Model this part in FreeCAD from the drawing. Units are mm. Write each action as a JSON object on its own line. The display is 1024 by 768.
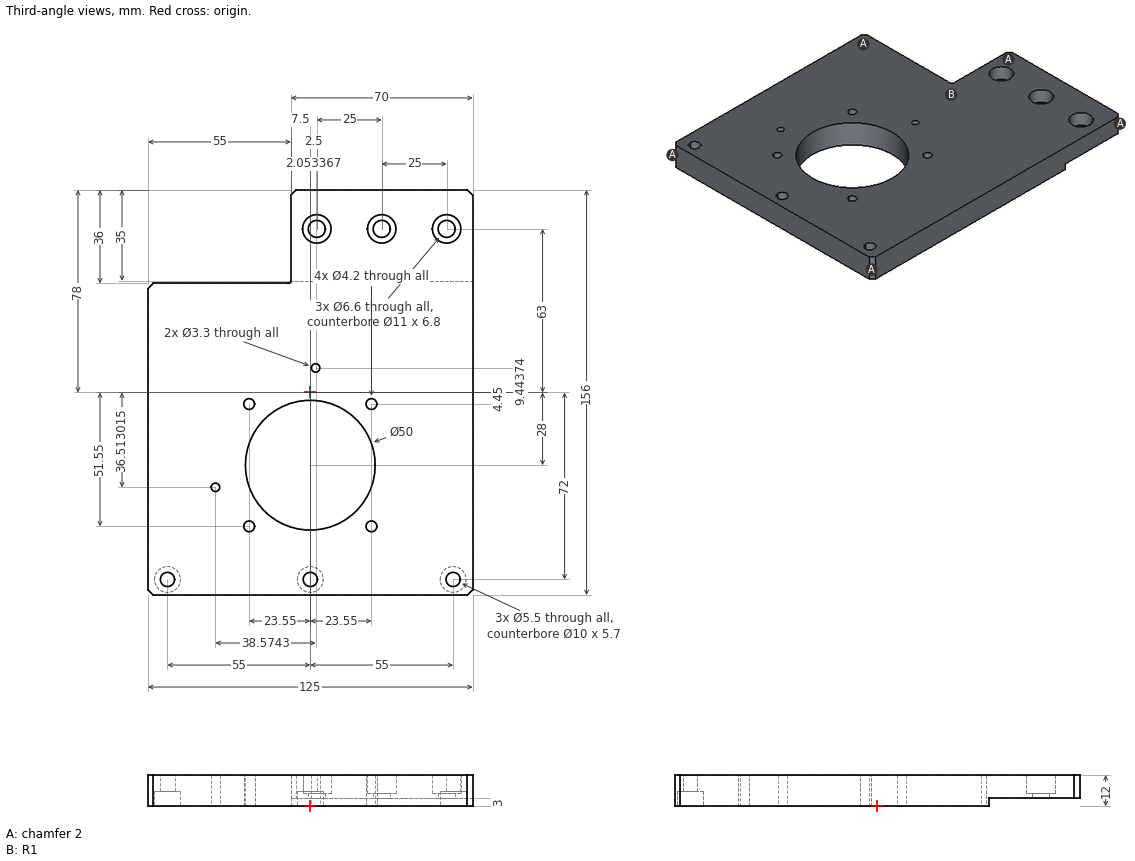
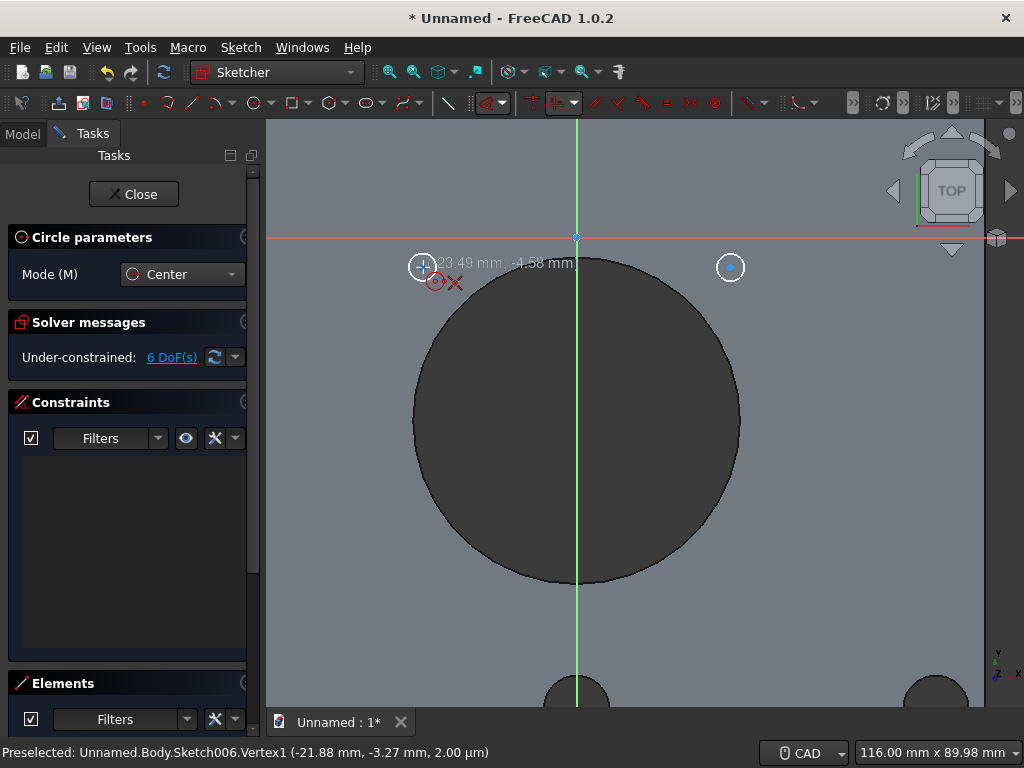
{"action": "scroll", "coordinate": [423, 575], "scroll_direction": "up", "scroll_amount": 3}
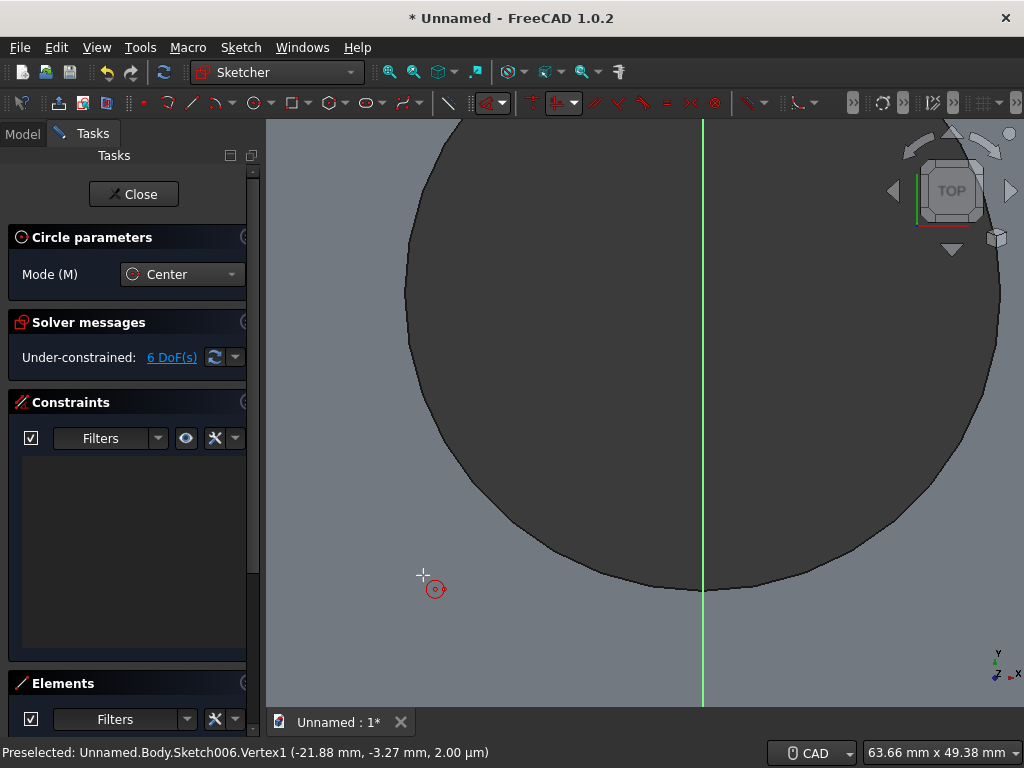
{"action": "left_click", "coordinate": [422, 574]}
{"action": "left_click", "coordinate": [440, 556]}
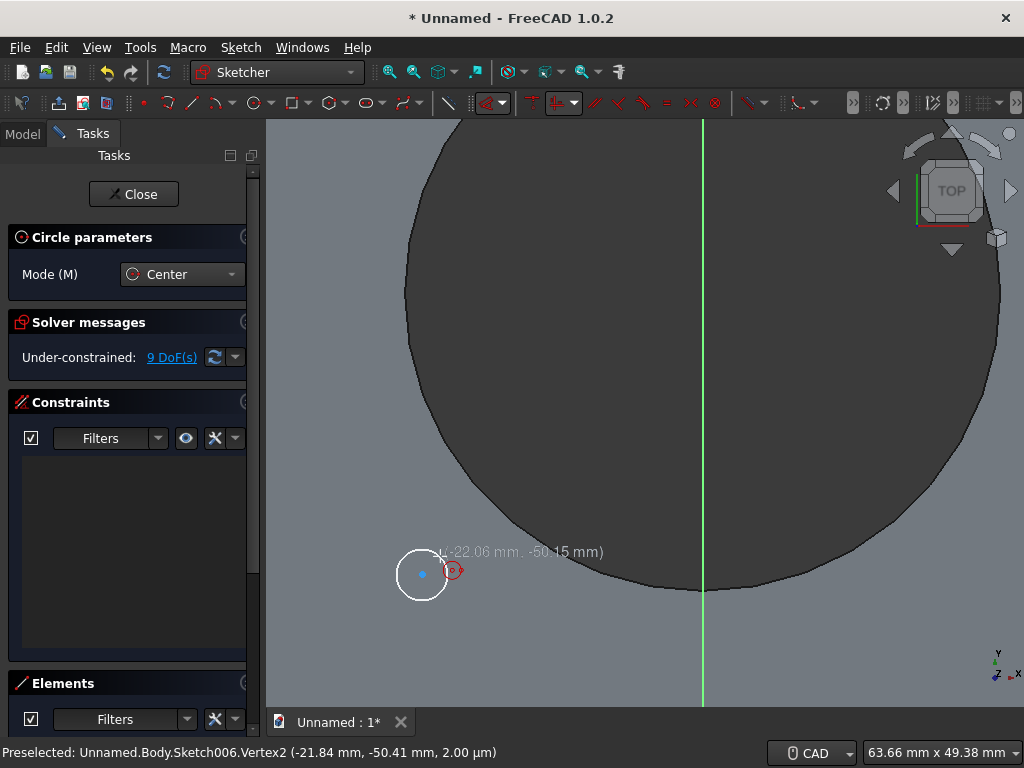
{"action": "scroll", "coordinate": [423, 576], "scroll_direction": "down", "scroll_amount": 3}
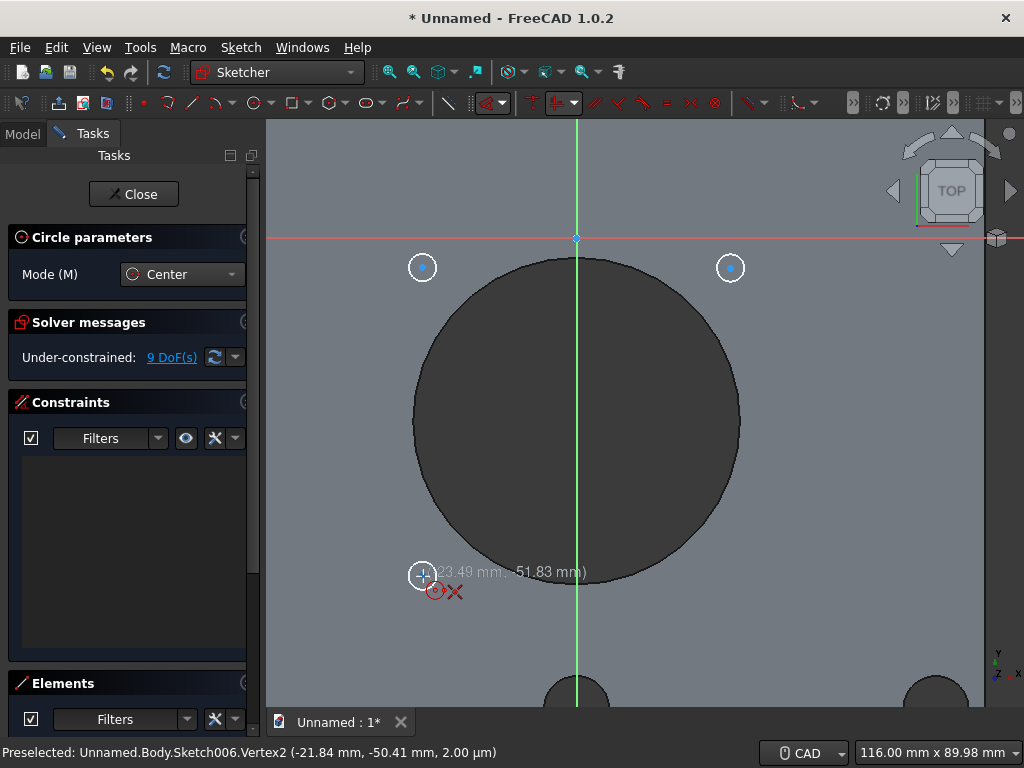
{"action": "scroll", "coordinate": [730, 575], "scroll_direction": "up", "scroll_amount": 3}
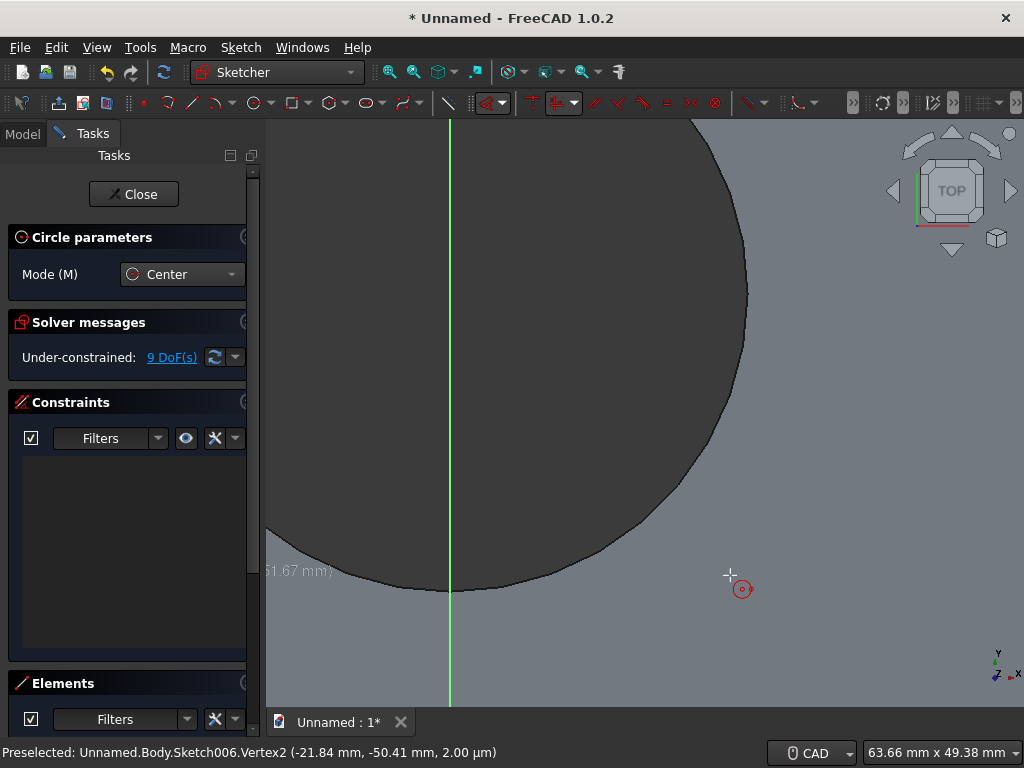
{"action": "left_click", "coordinate": [730, 574]}
{"action": "left_click", "coordinate": [748, 557]}
{"action": "key", "text": "Escape"}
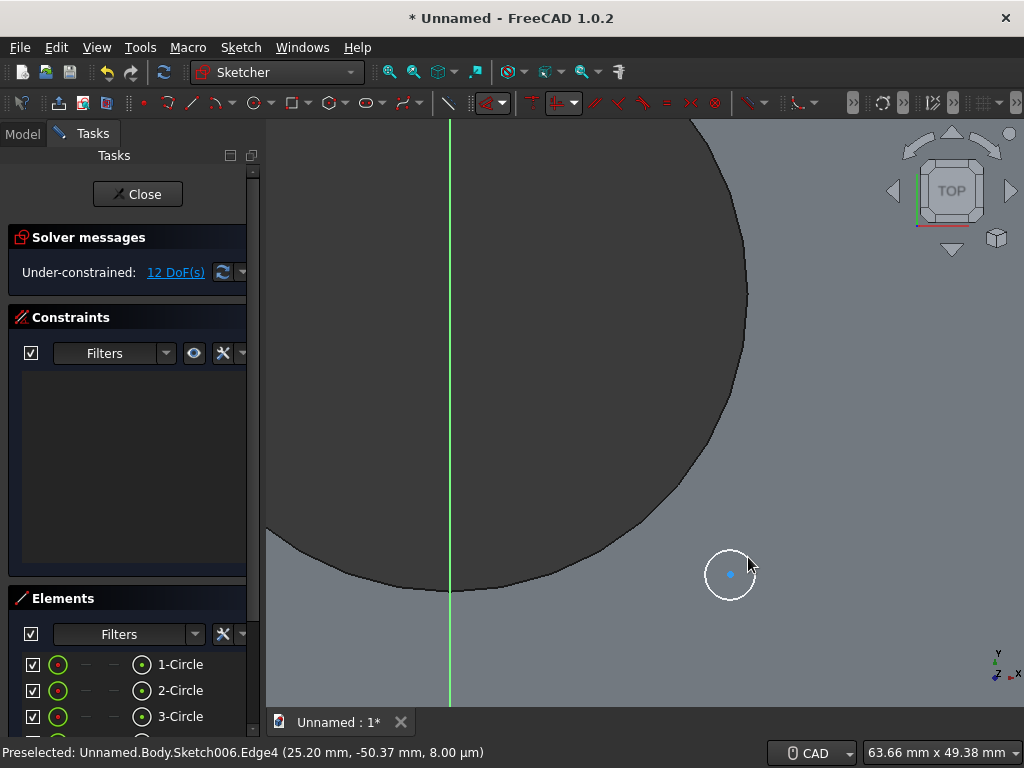
{"action": "scroll", "coordinate": [730, 575], "scroll_direction": "down", "scroll_amount": 3}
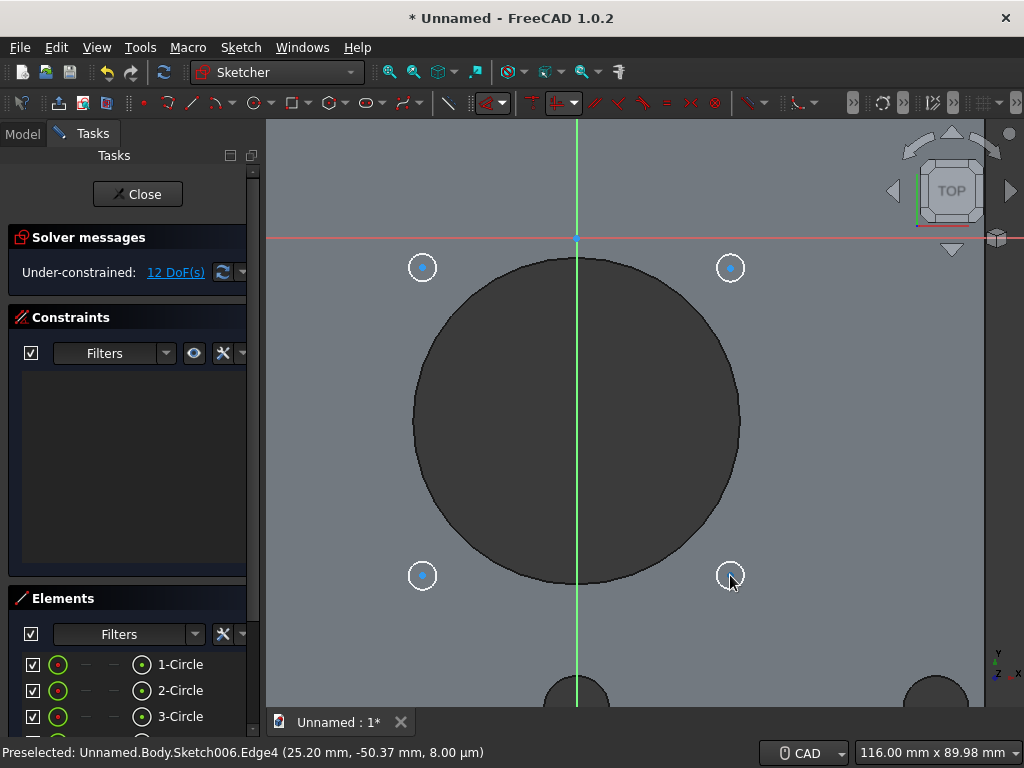
{"action": "left_click", "coordinate": [740, 258]}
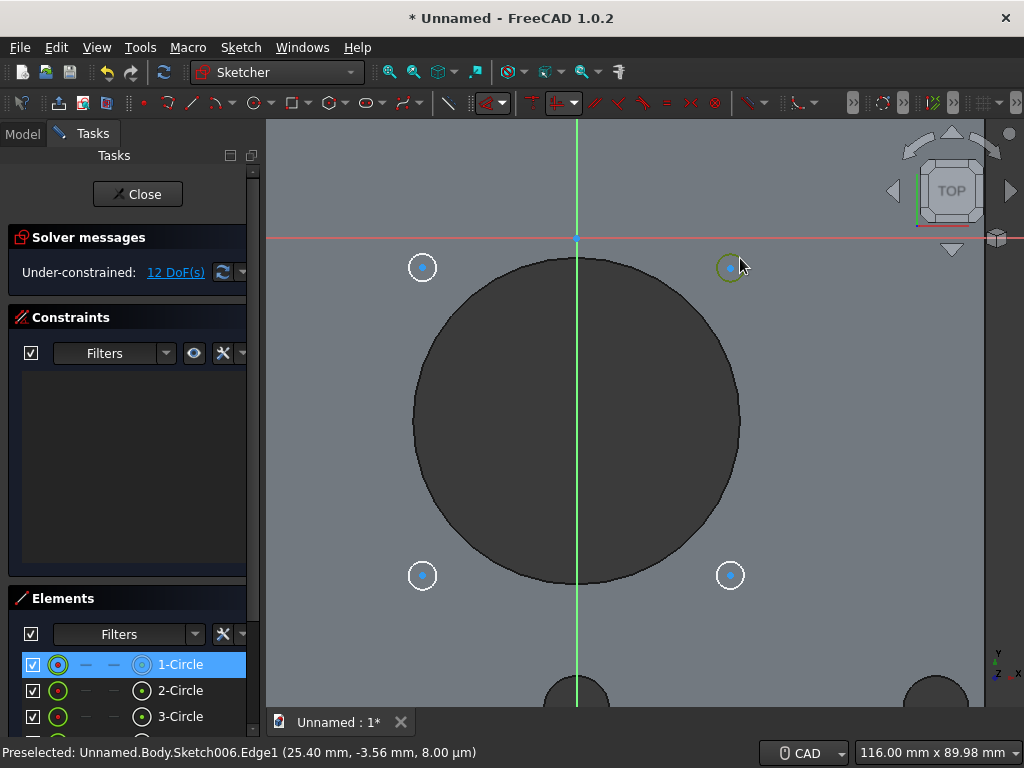
{"action": "left_click", "coordinate": [432, 258]}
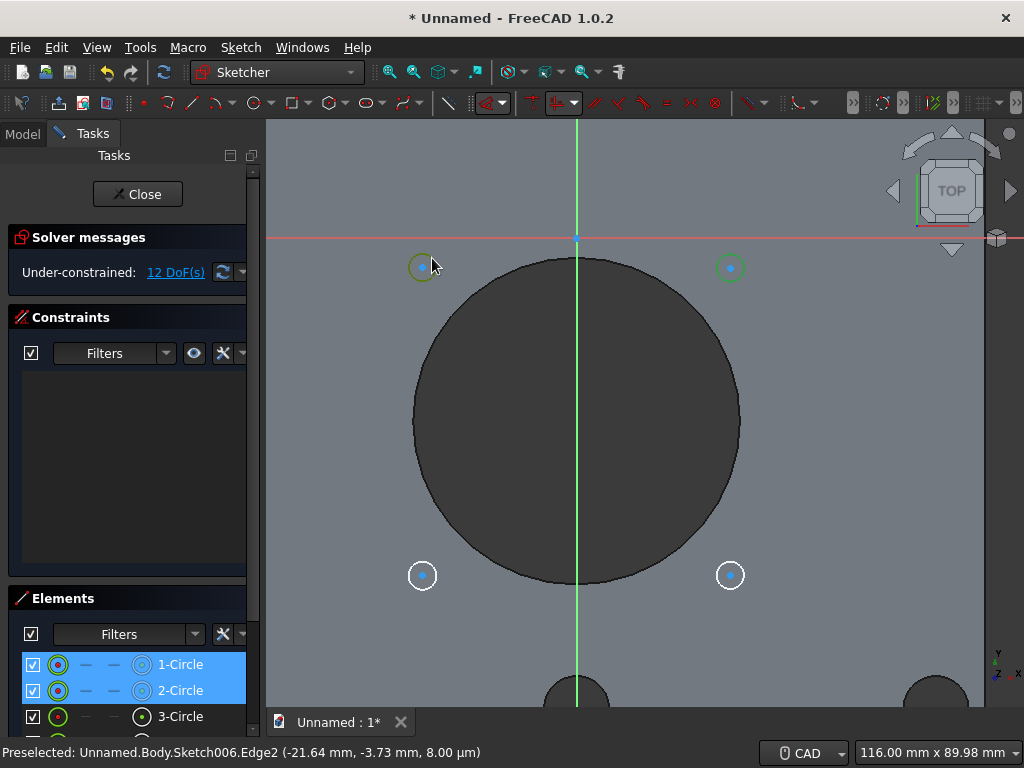
{"action": "left_click", "coordinate": [432, 566]}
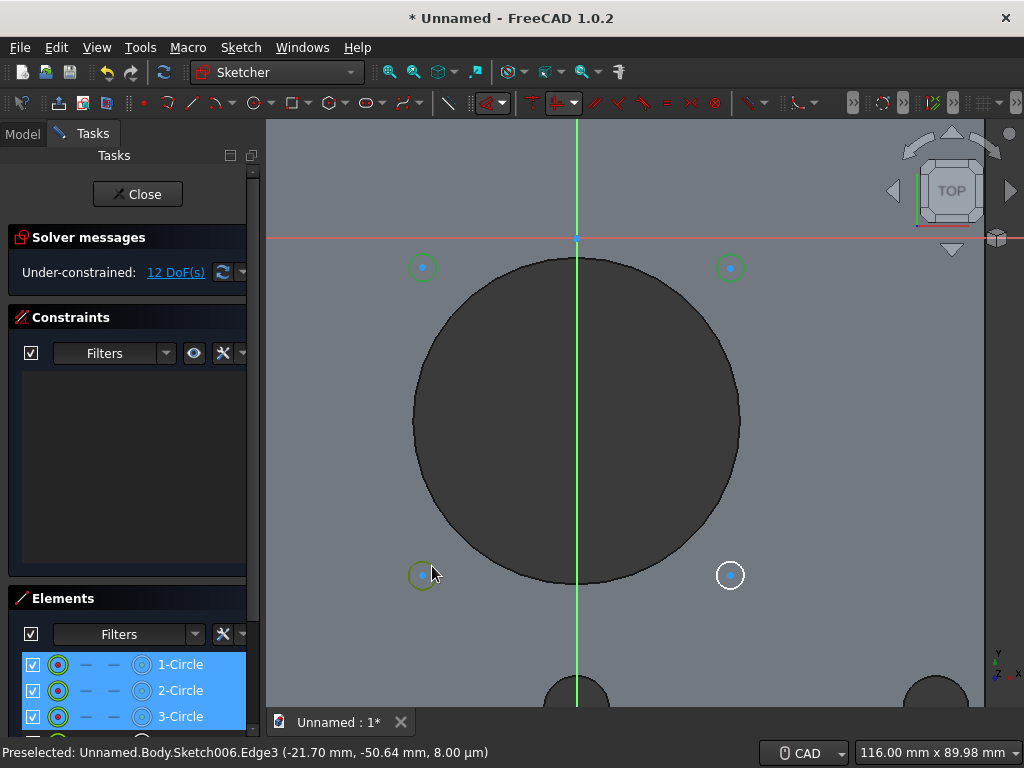
{"action": "left_click", "coordinate": [740, 566]}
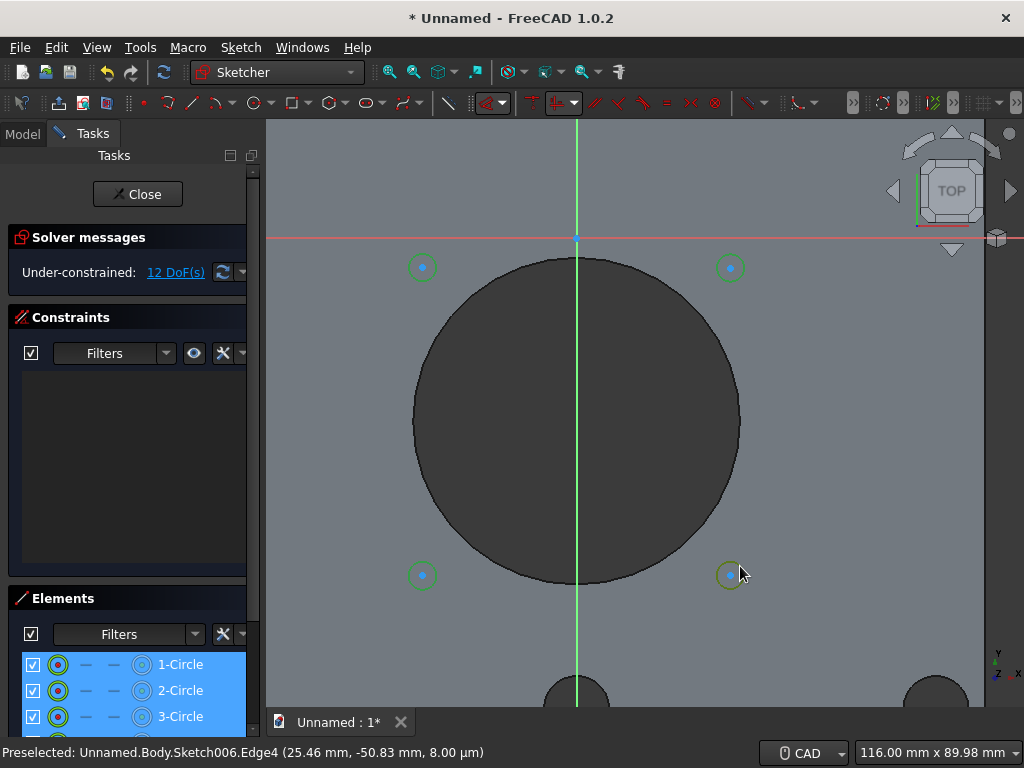
{"action": "left_click", "coordinate": [668, 104]}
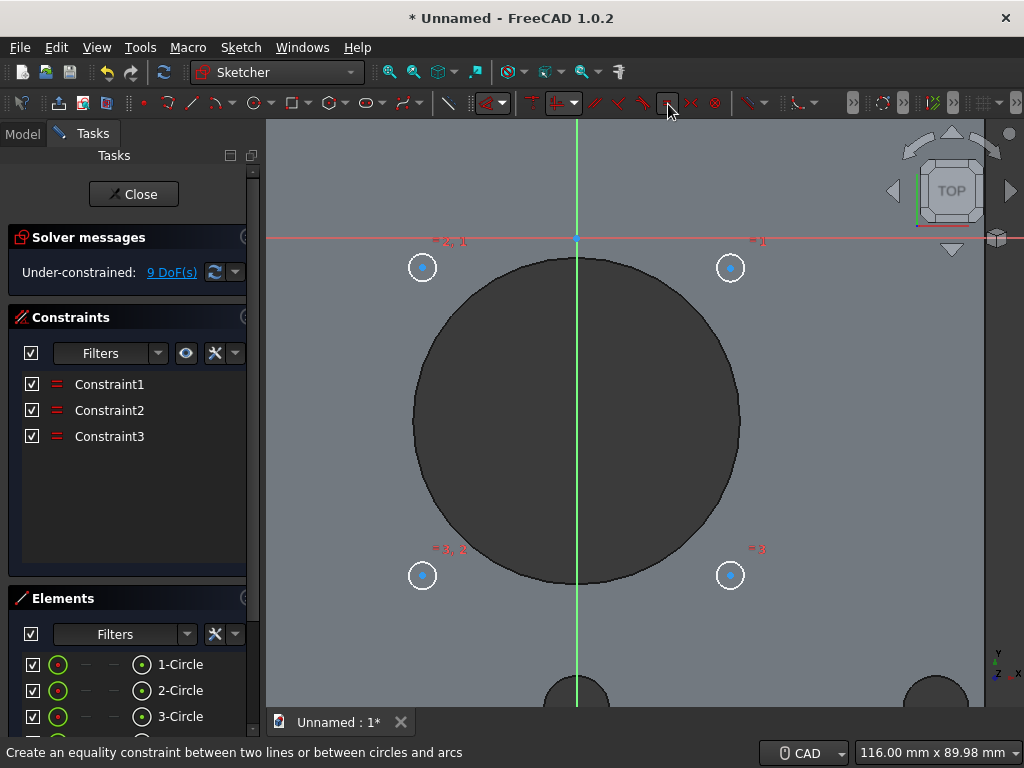
{"action": "left_click", "coordinate": [731, 268]}